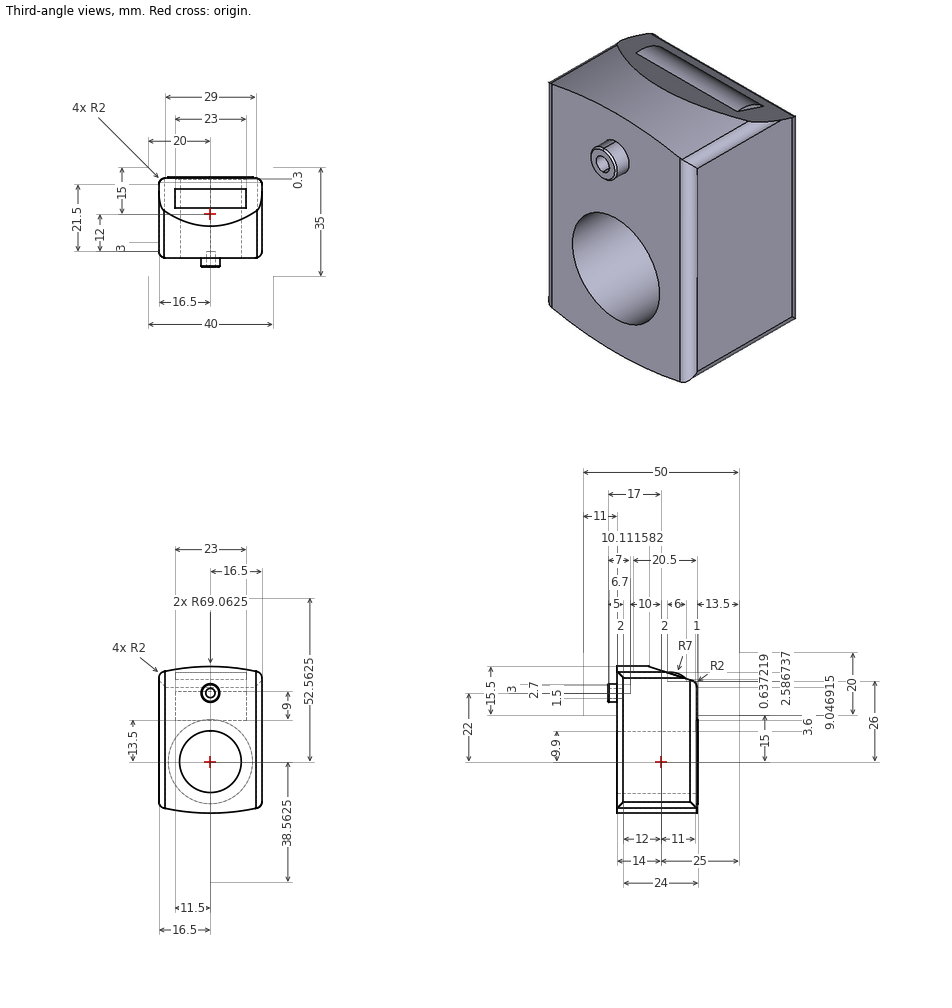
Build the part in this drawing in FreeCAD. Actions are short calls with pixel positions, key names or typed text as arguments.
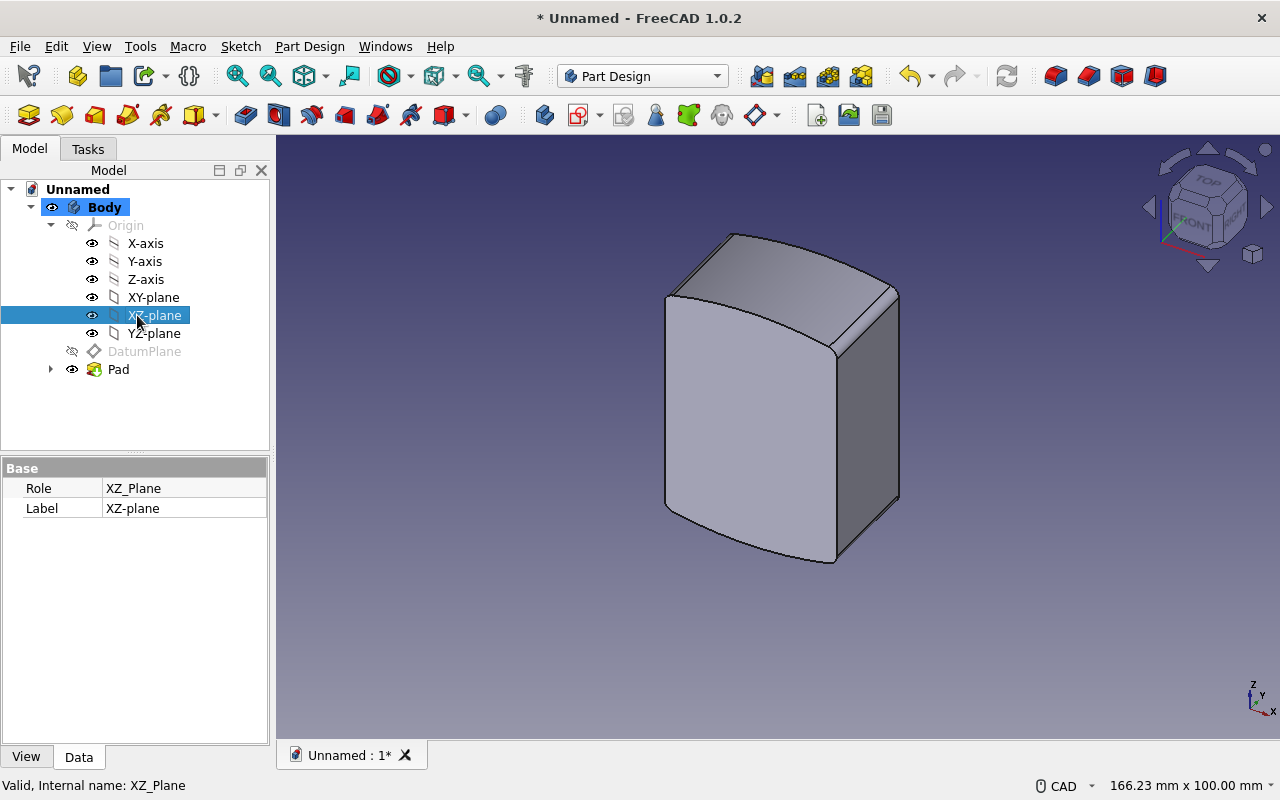
click(754, 116)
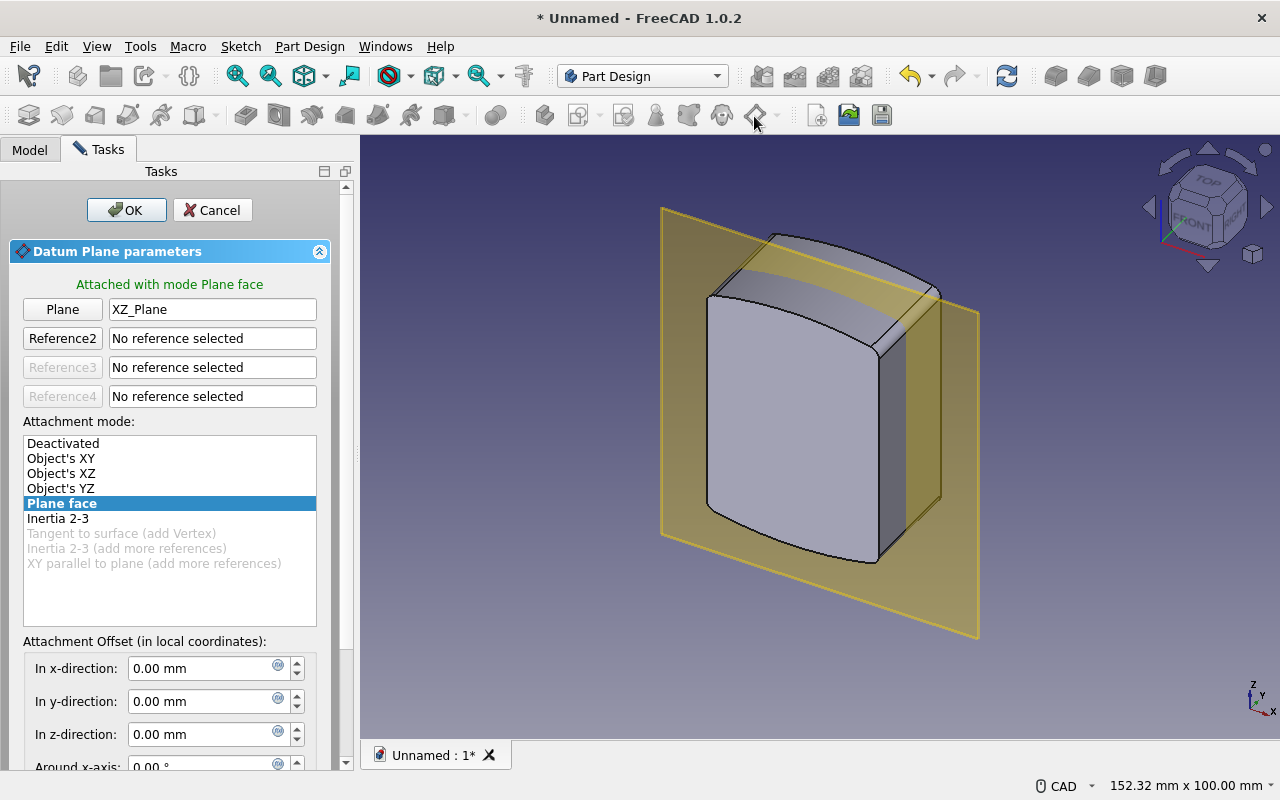
triple_click(210, 734)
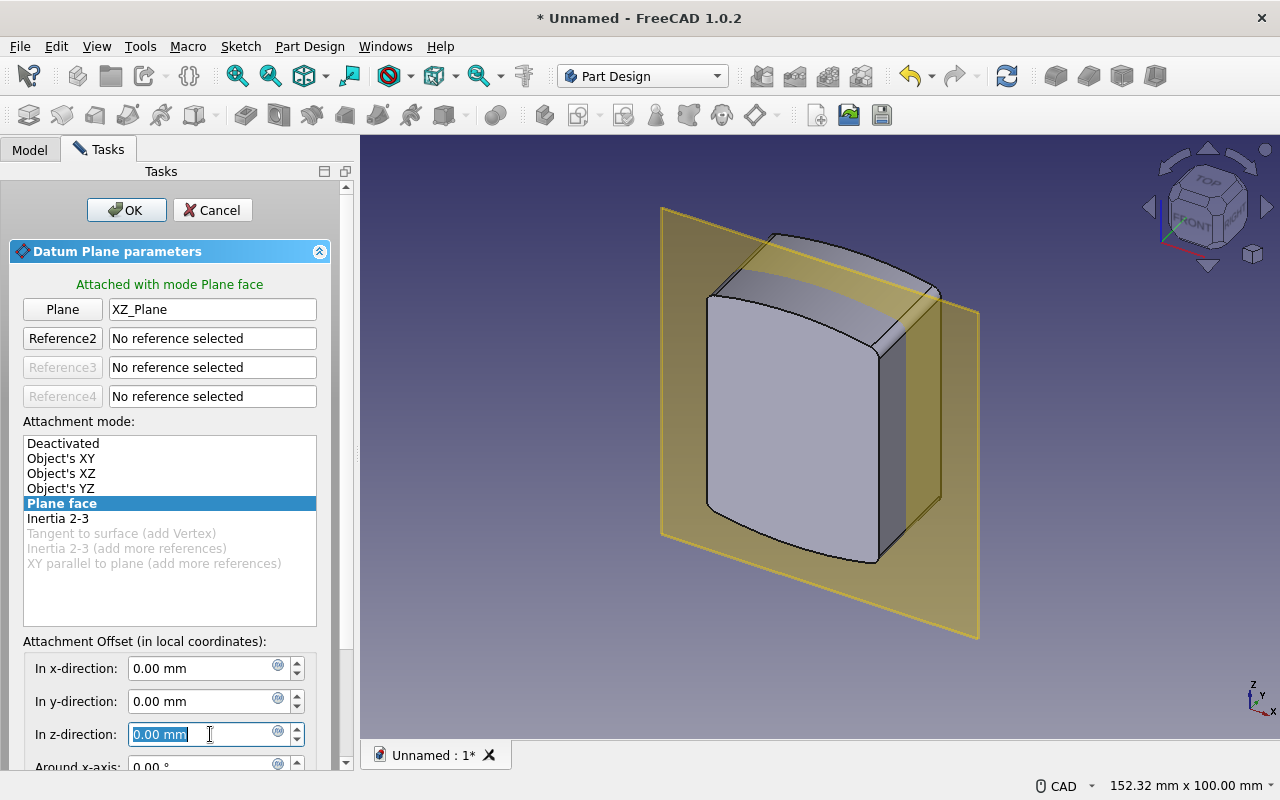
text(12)
key(Tab)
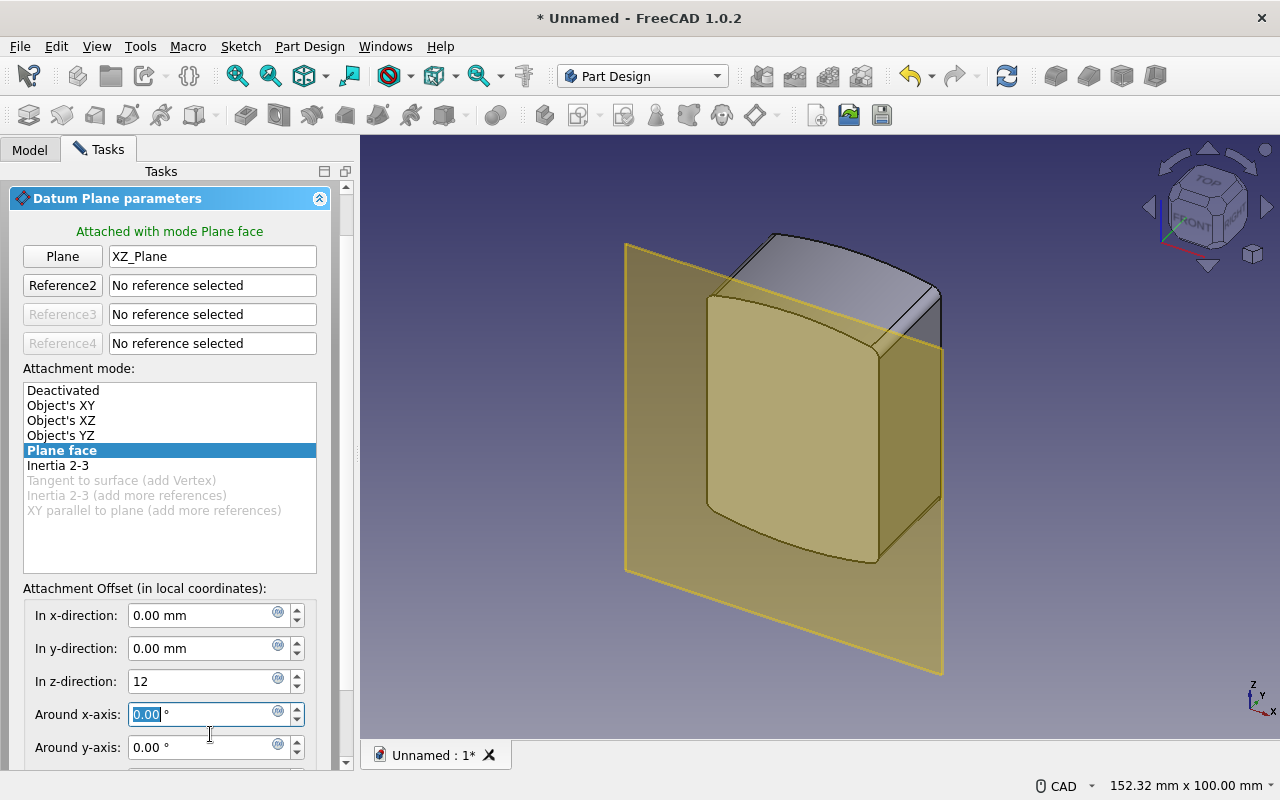
scroll(346, 476, up, 2)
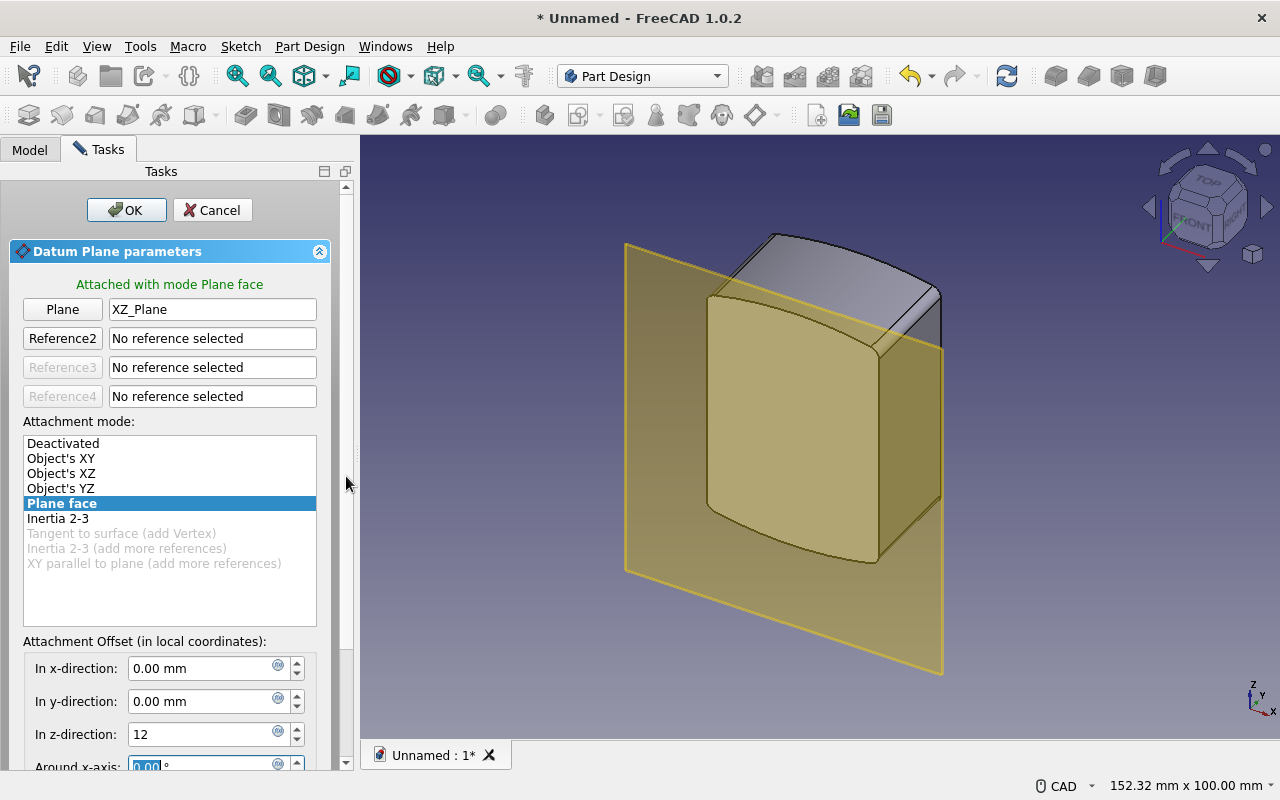
click(127, 210)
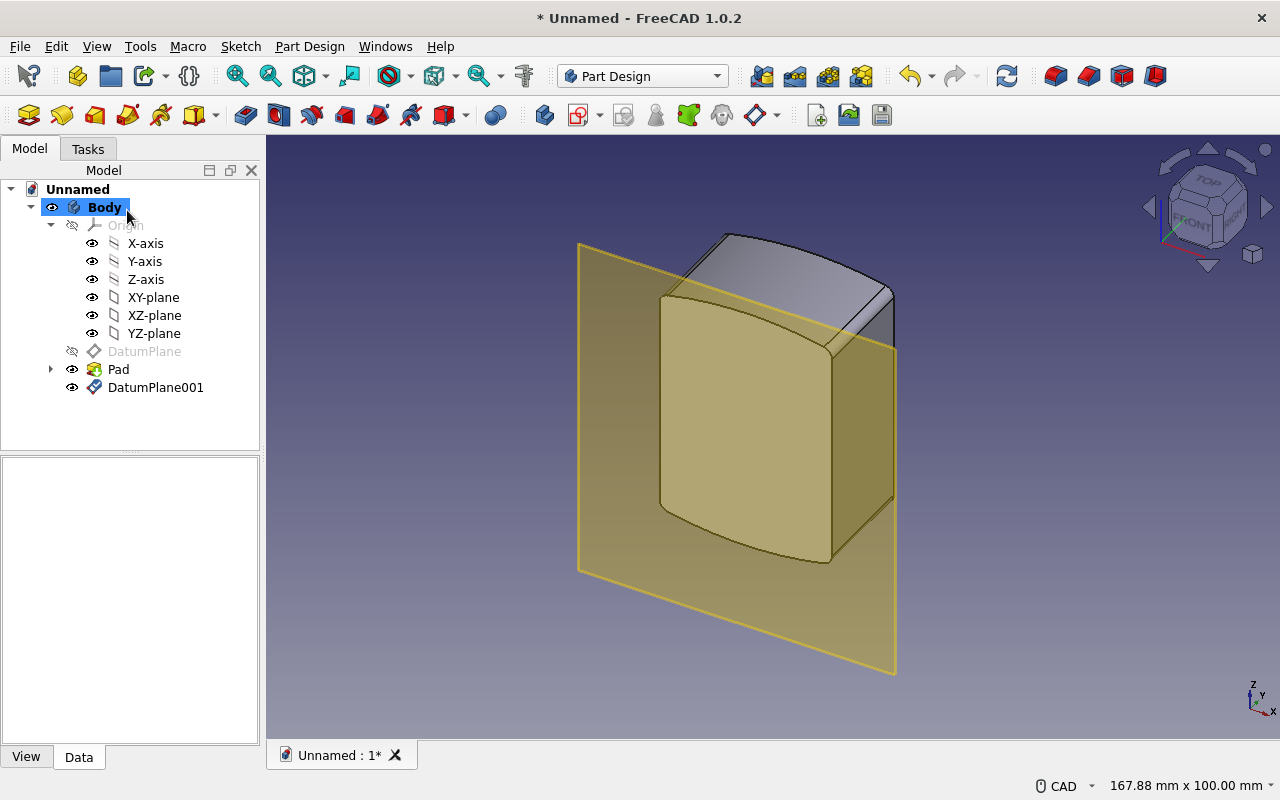
click(117, 387)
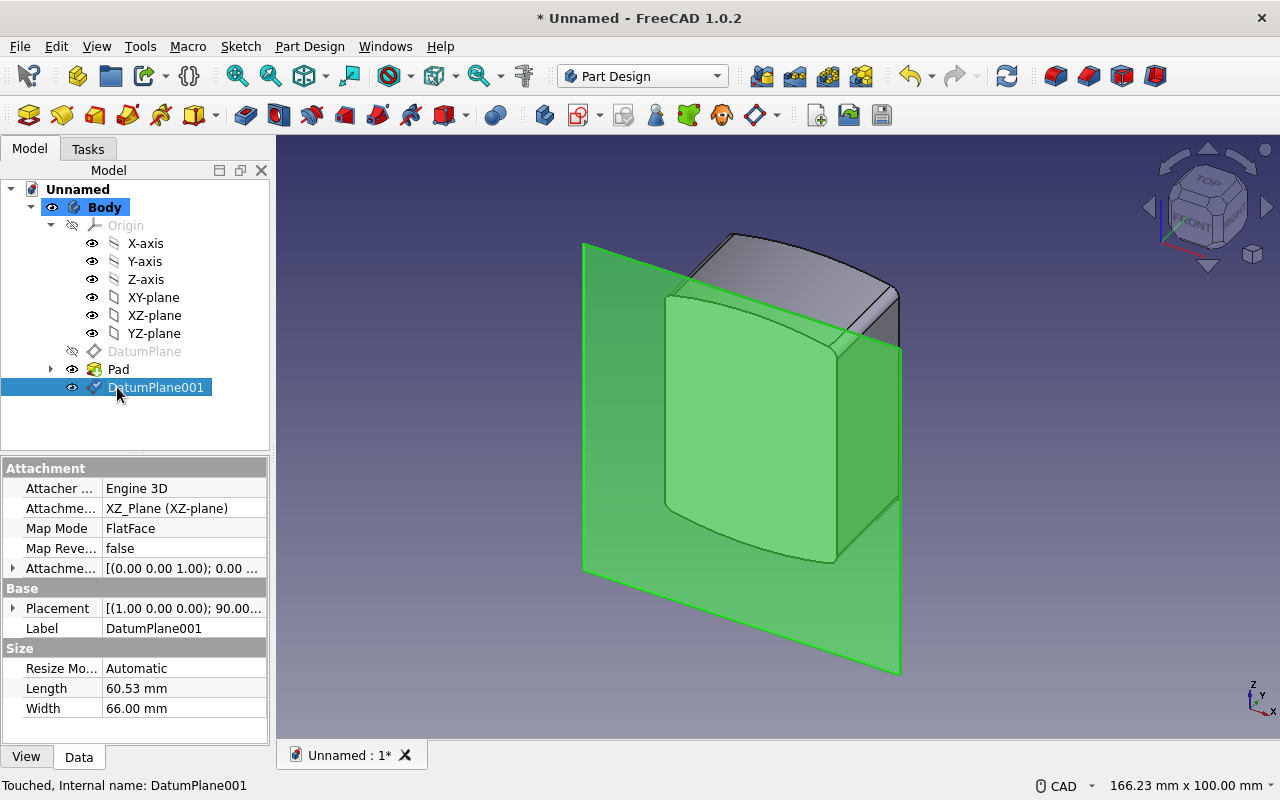
click(578, 116)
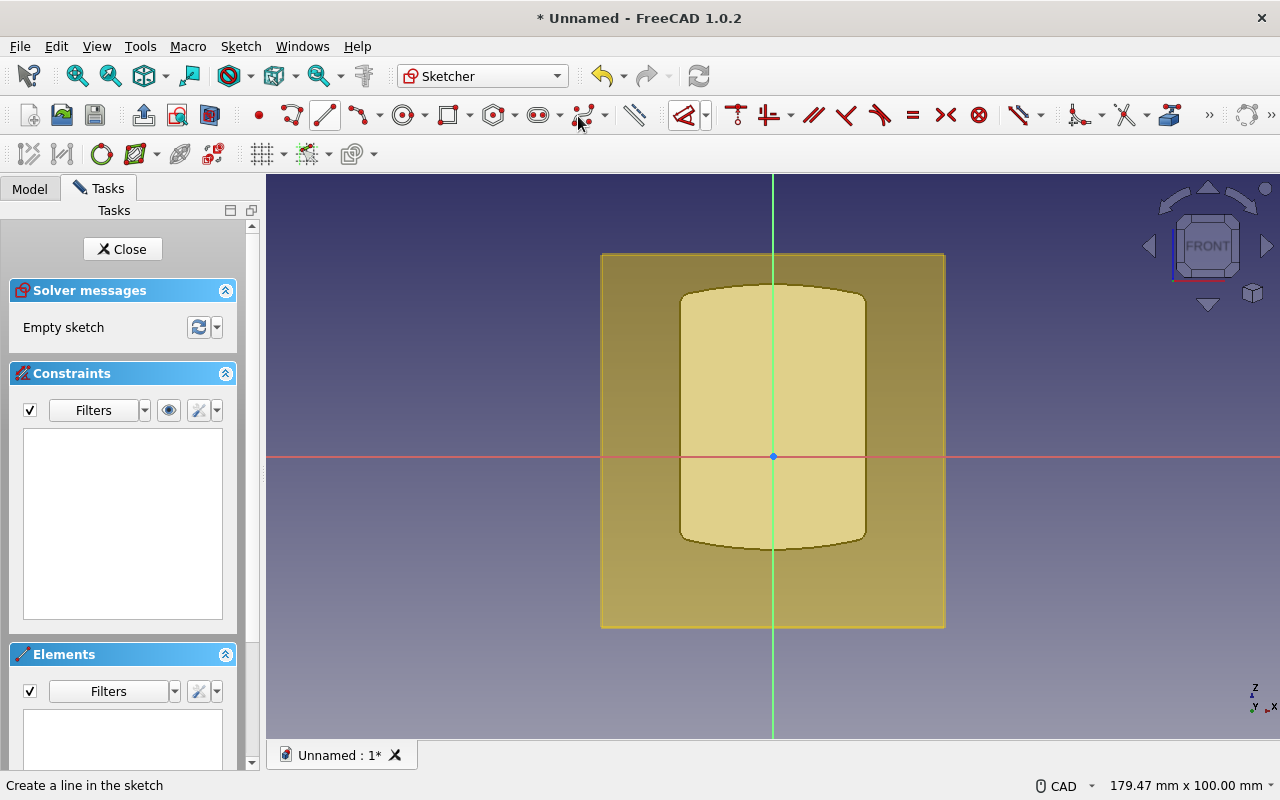
scroll(912, 337, up, 2)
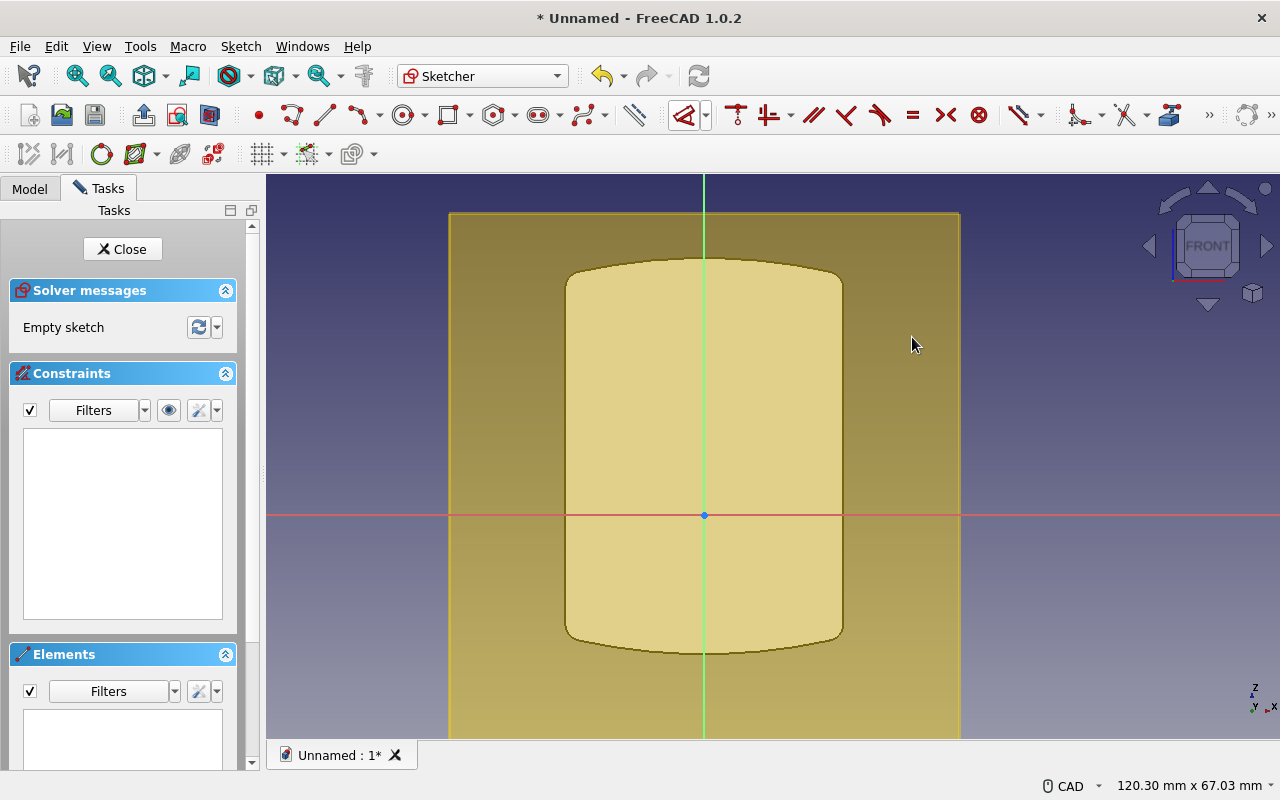
click(325, 116)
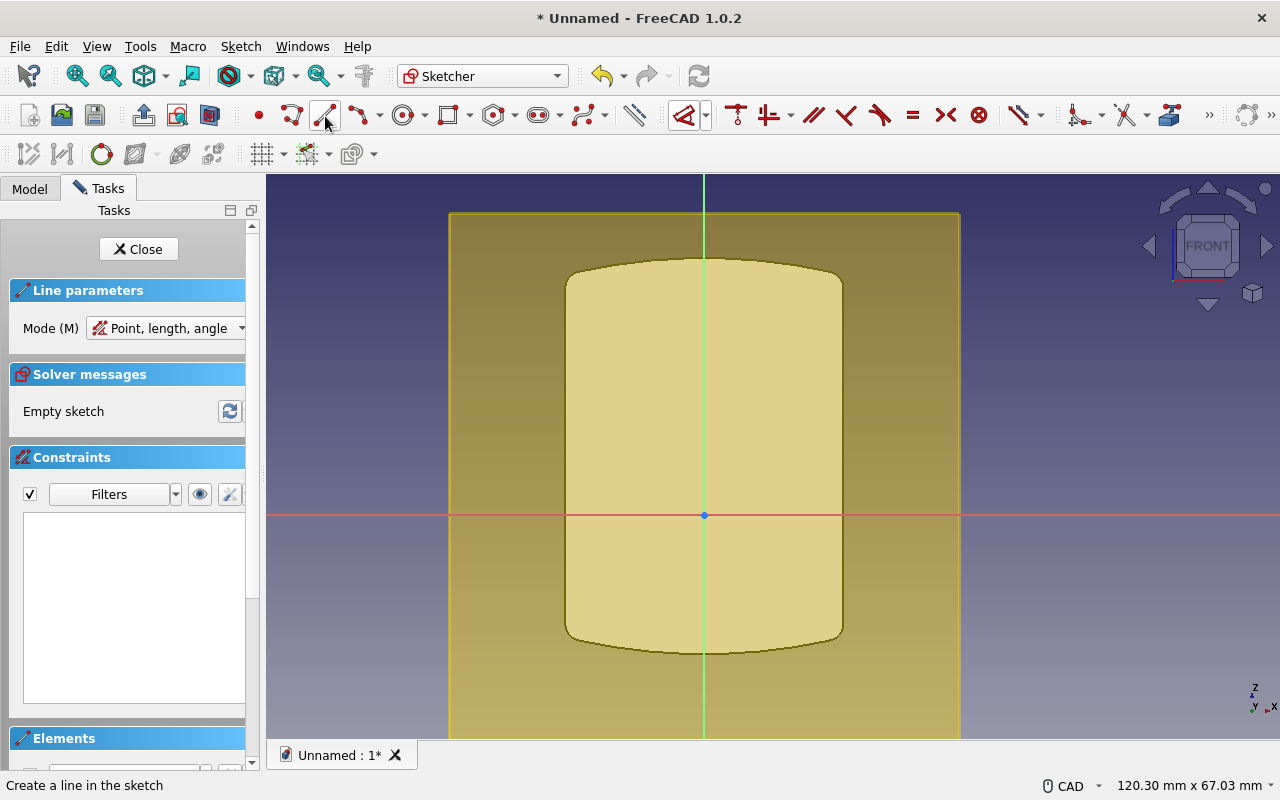
click(565, 624)
click(565, 288)